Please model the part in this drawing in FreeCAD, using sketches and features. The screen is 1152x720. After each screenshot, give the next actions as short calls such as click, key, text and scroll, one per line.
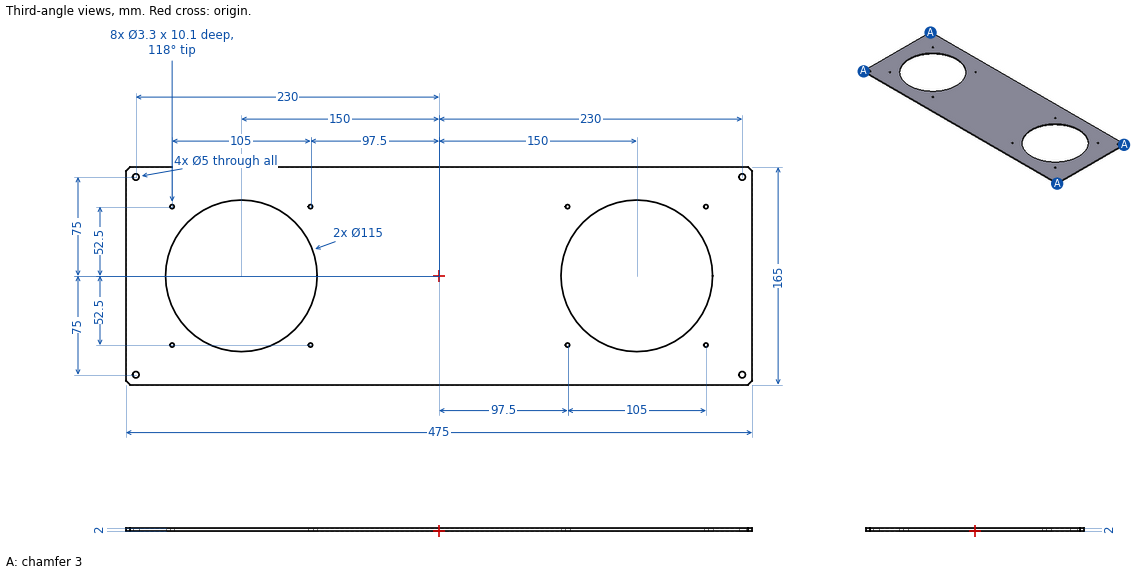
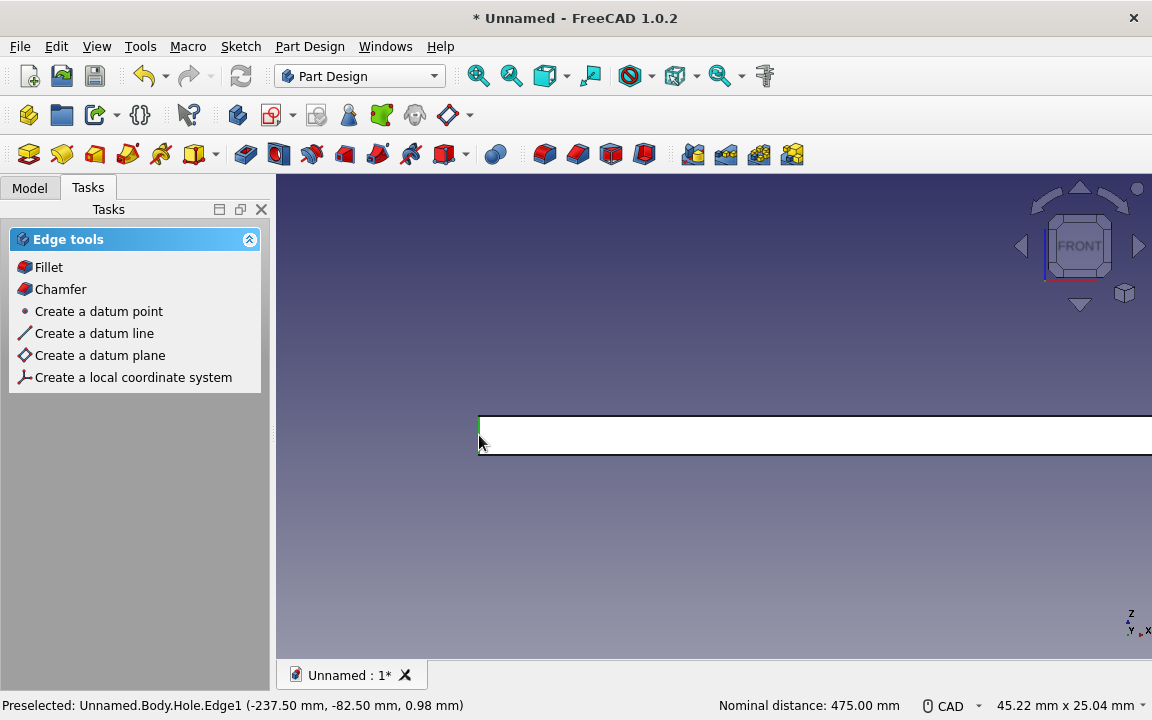
key(v)
key(f)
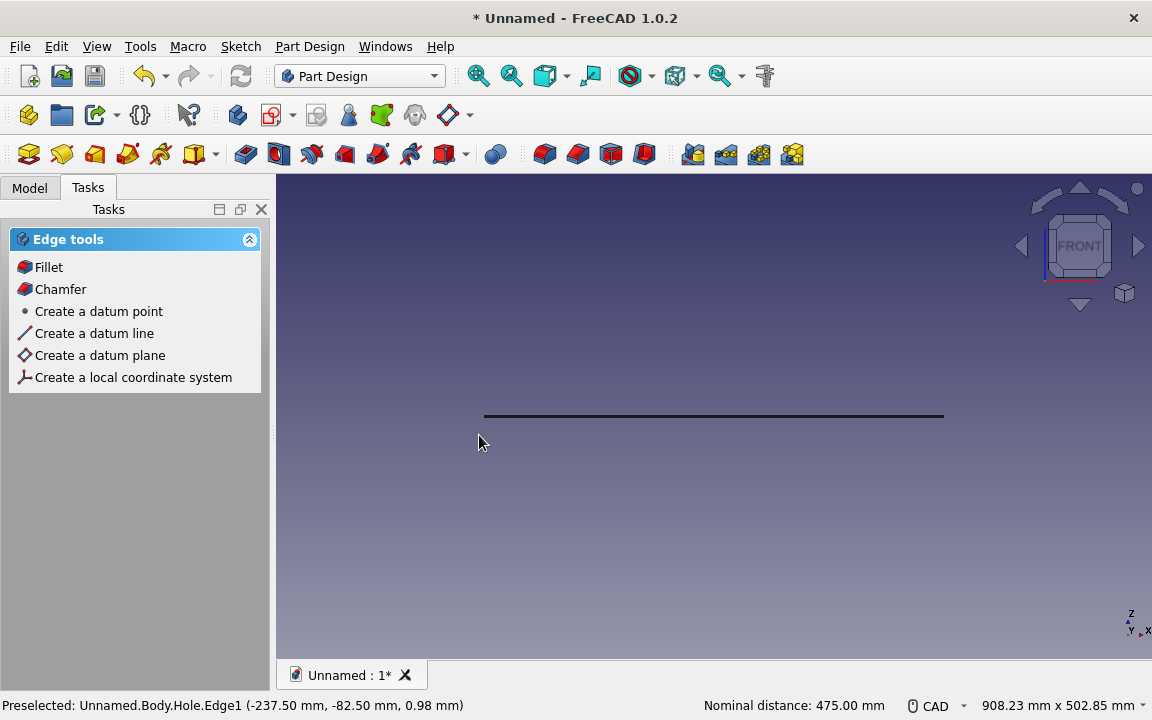
key(3)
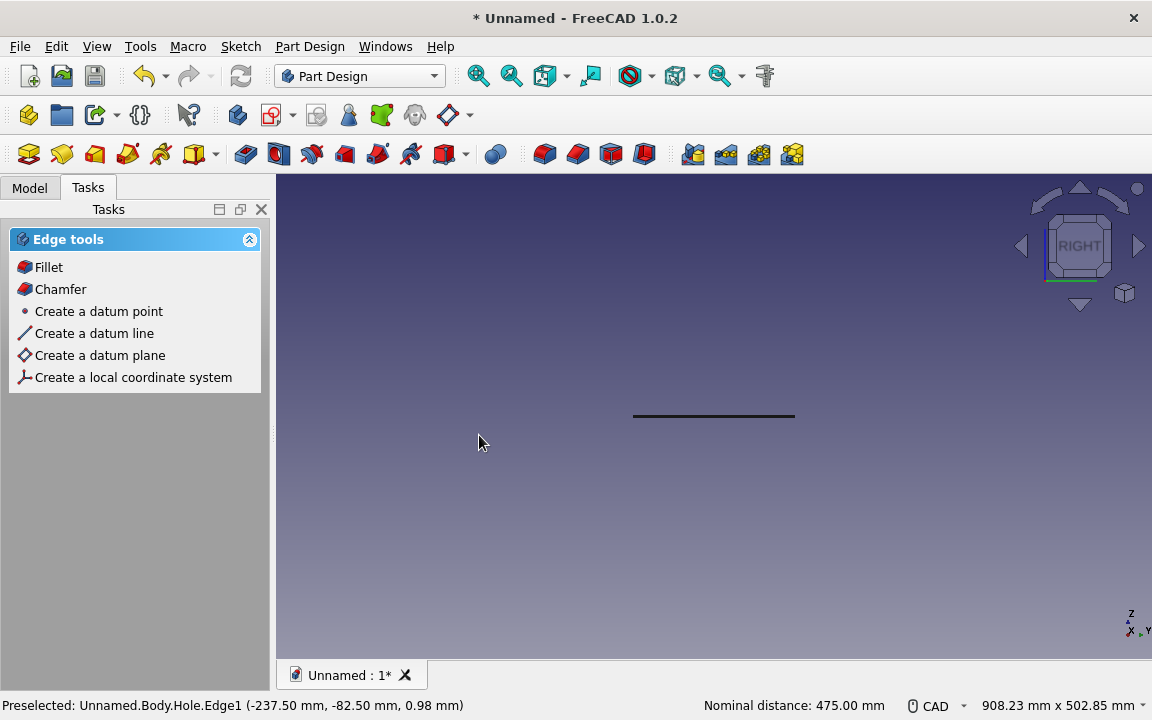
key(v)
key(f)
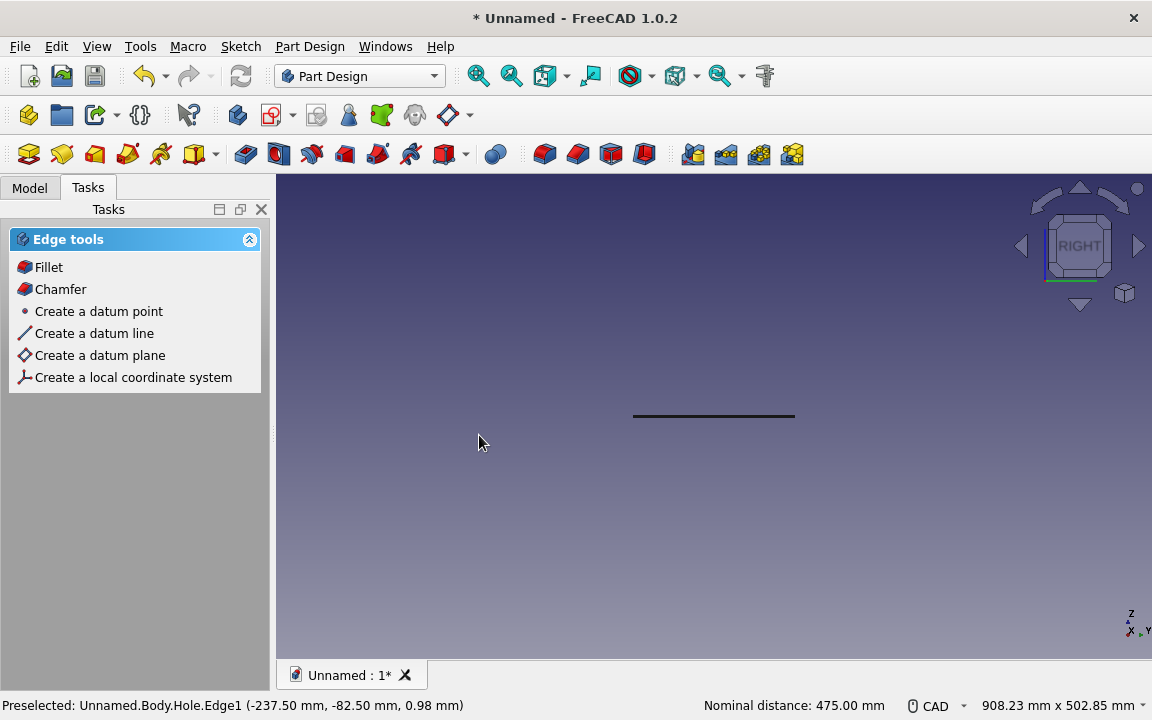
scroll(794, 415, up, 15)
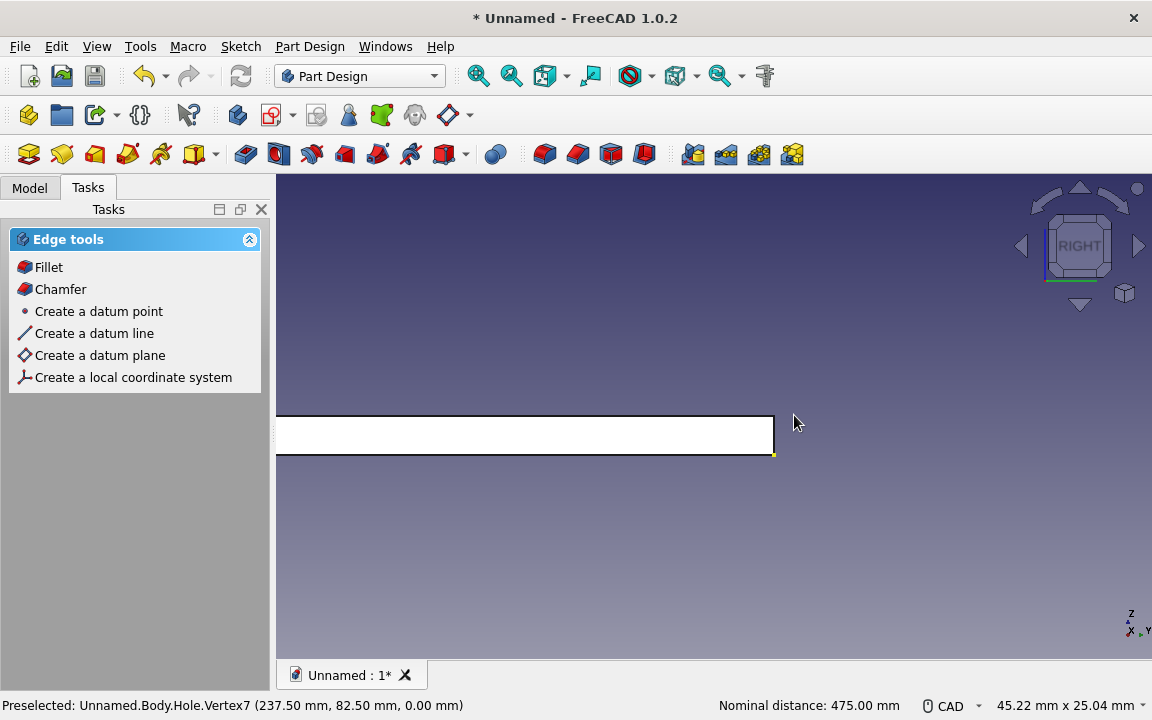
click(774, 435, ctrl)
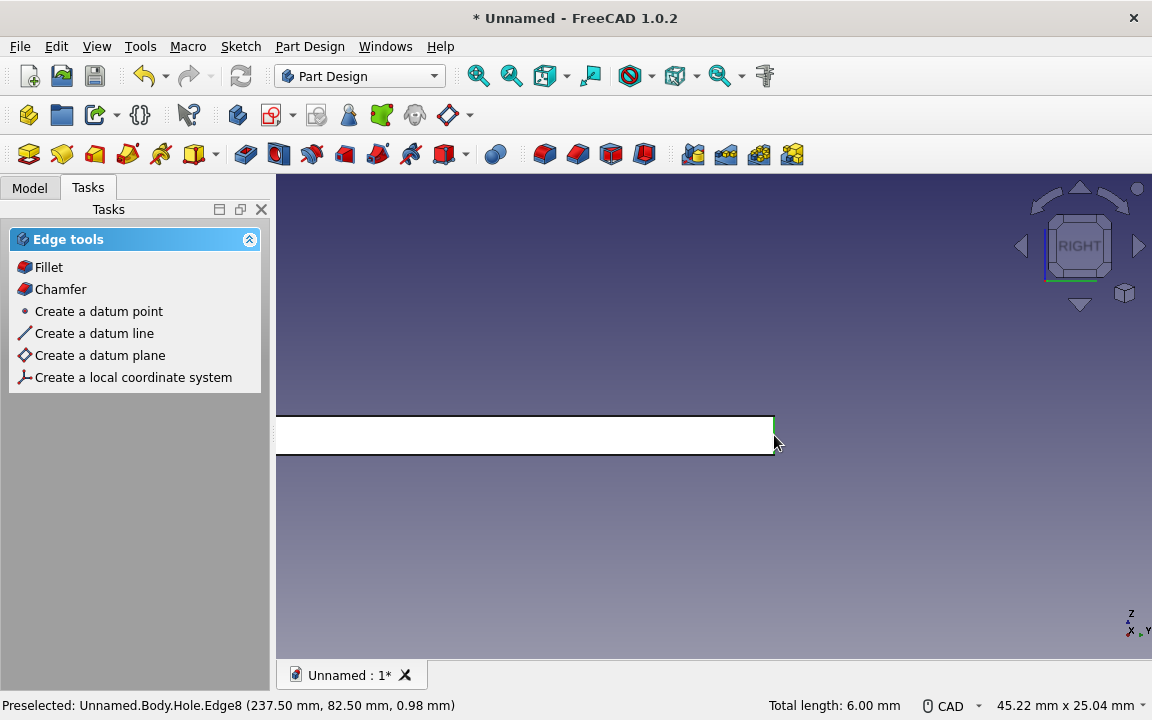
click(479, 76)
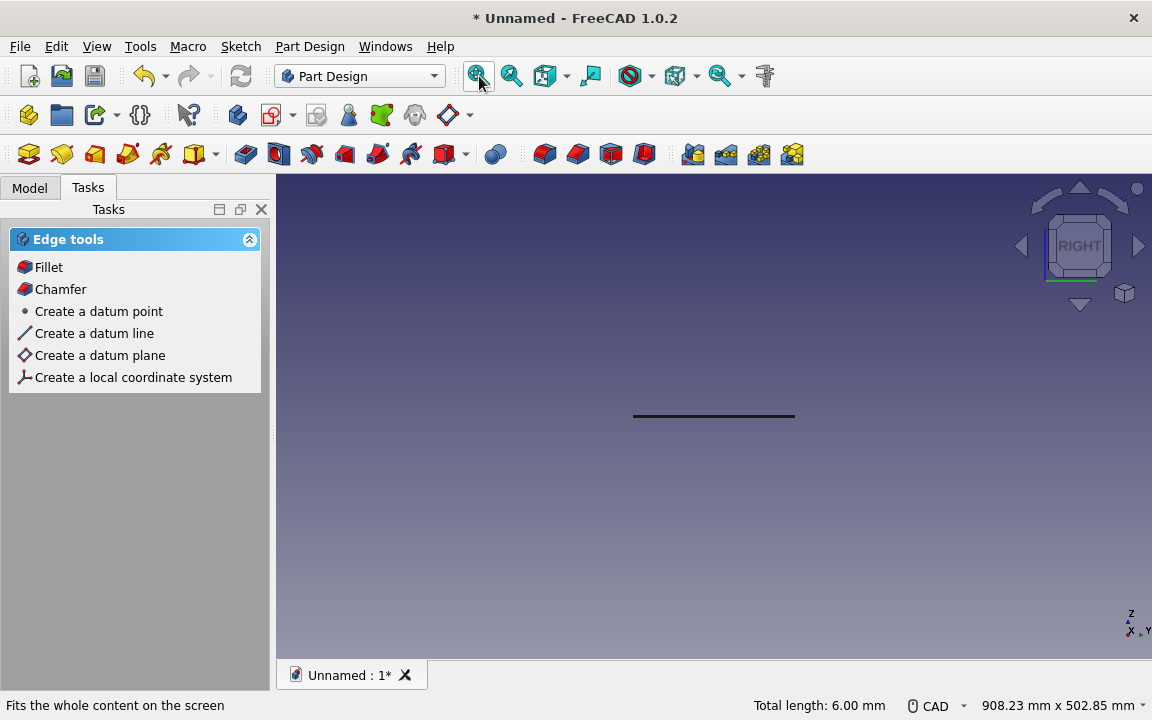
key(5)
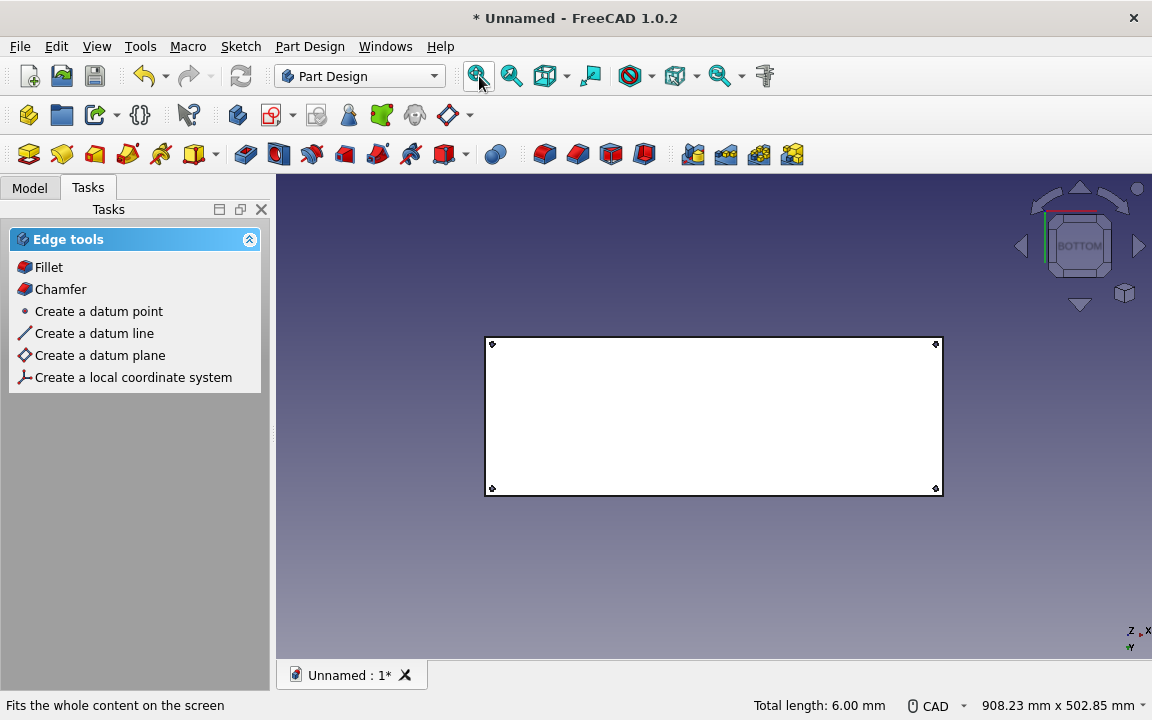
scroll(485, 495, up, 15)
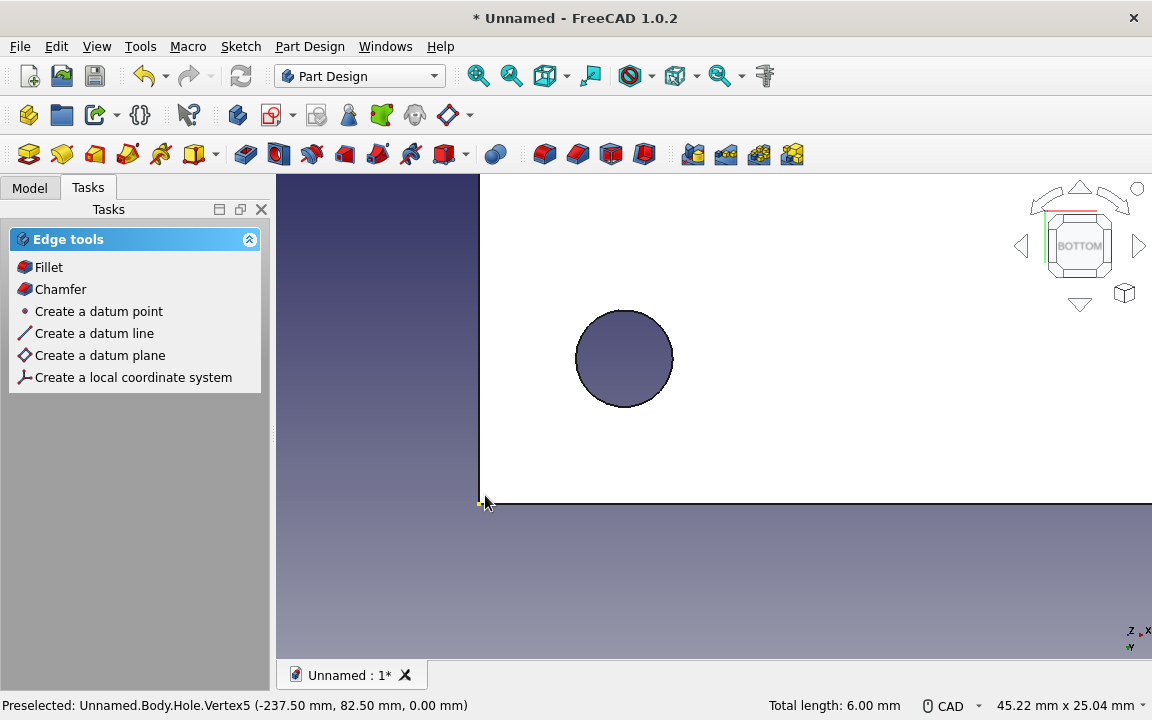
click(479, 76)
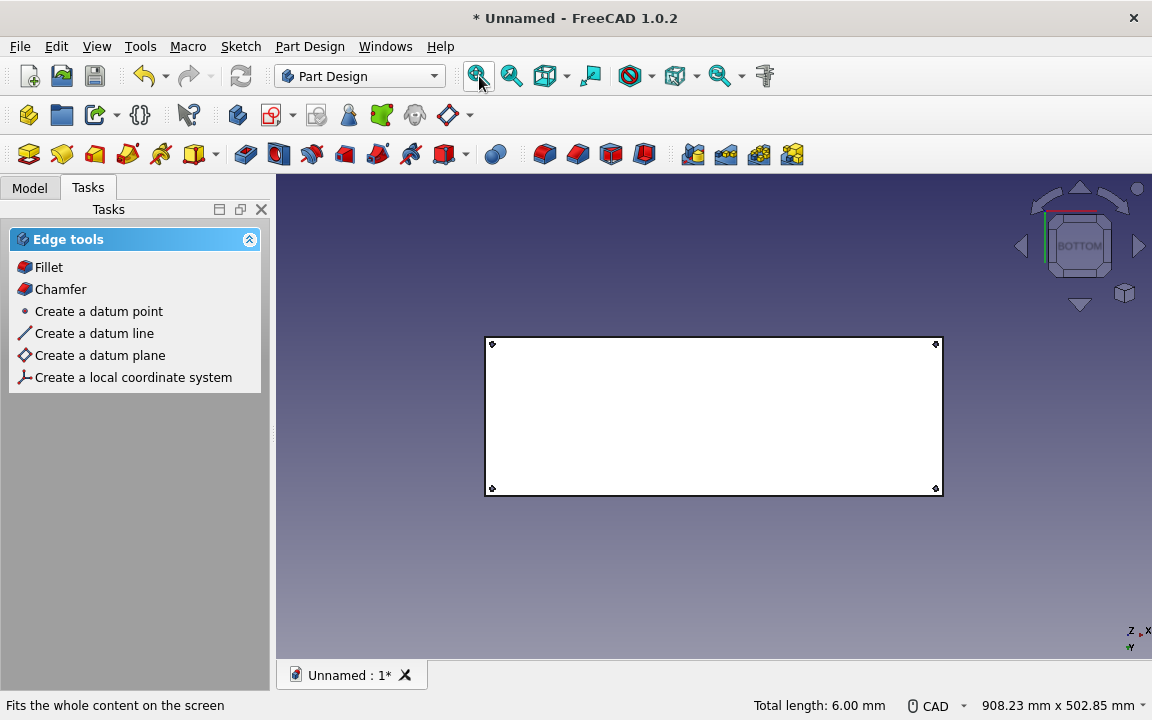
key(4)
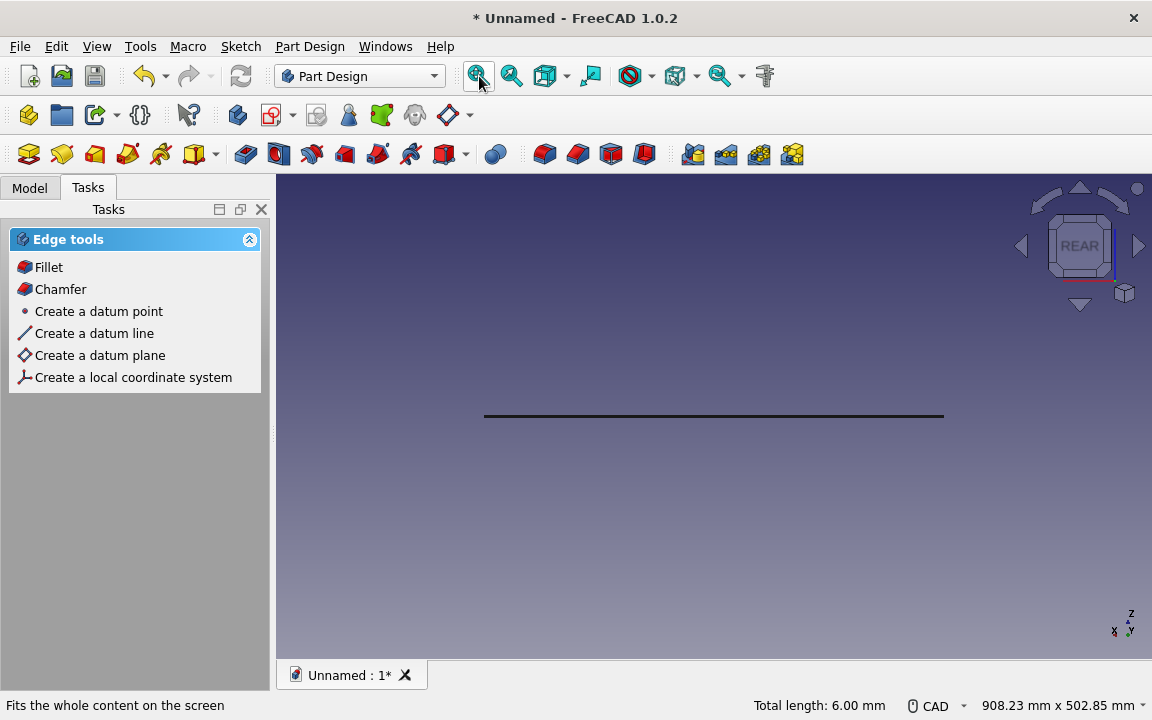
scroll(943, 415, up, 15)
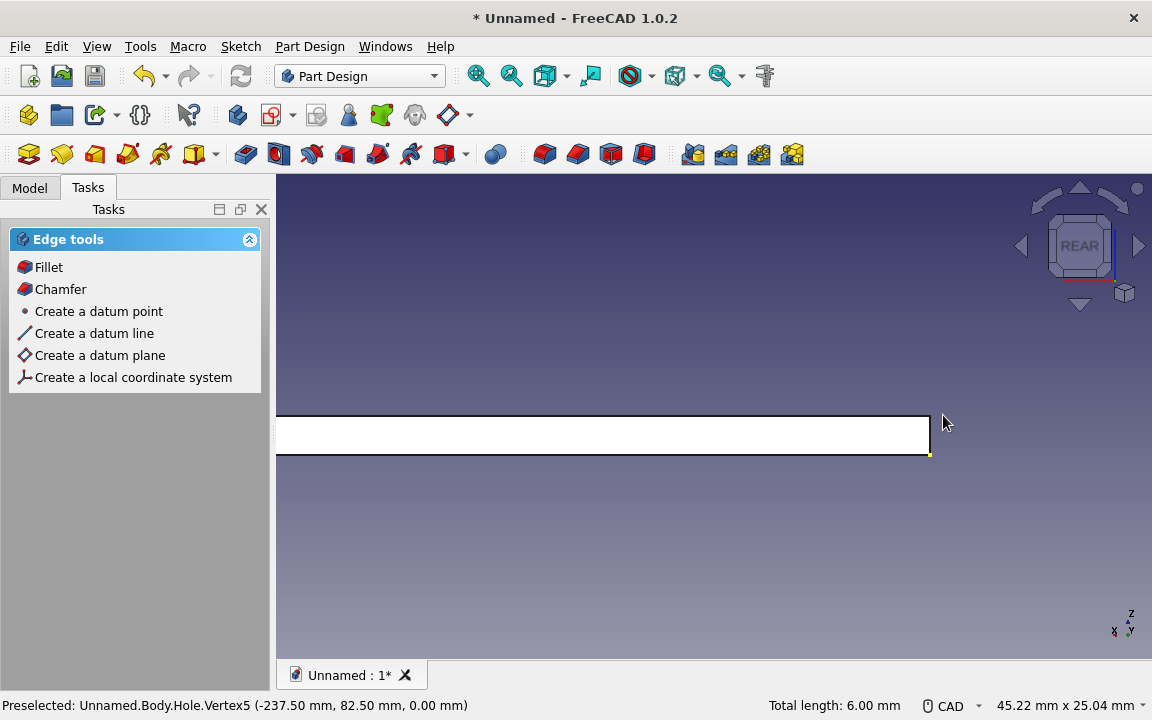
click(930, 435, ctrl)